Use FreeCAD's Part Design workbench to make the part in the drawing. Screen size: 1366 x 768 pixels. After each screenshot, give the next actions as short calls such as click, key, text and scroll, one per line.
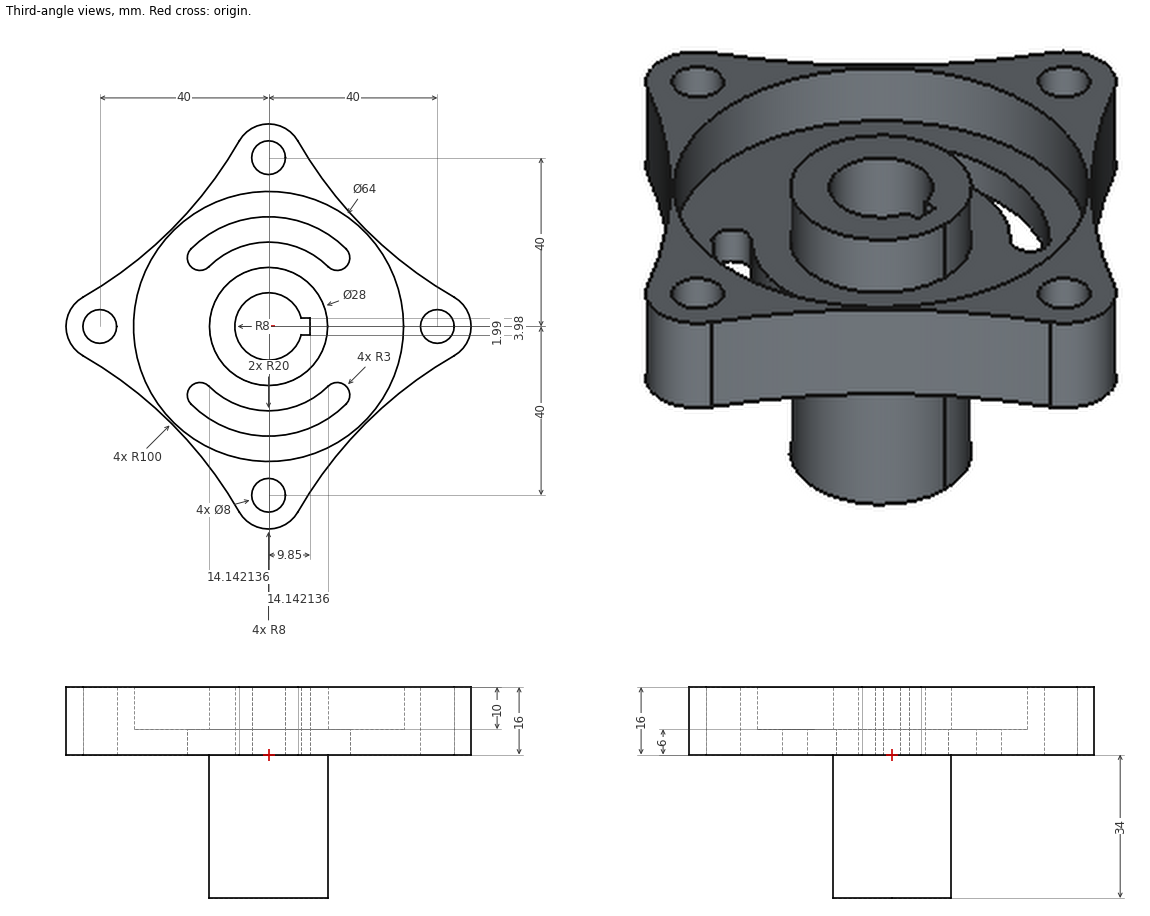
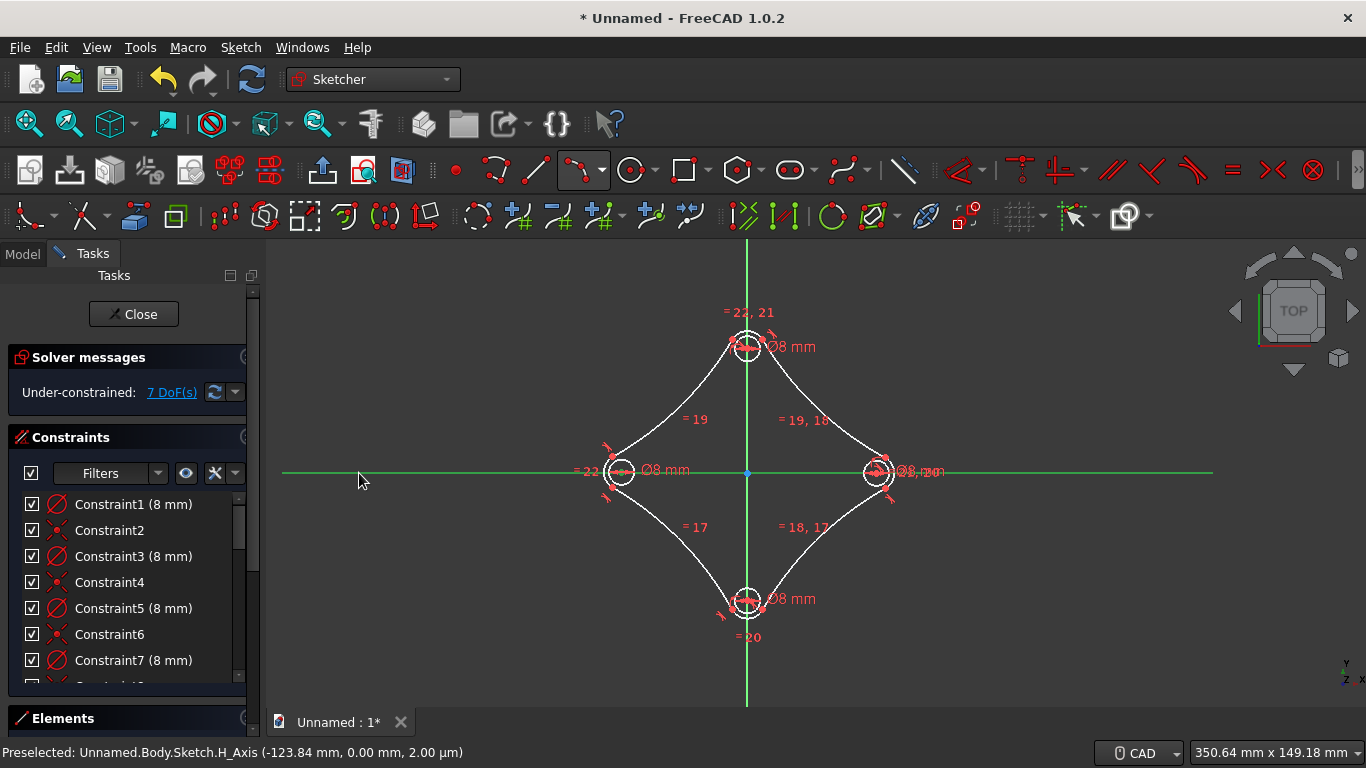
click(1020, 170)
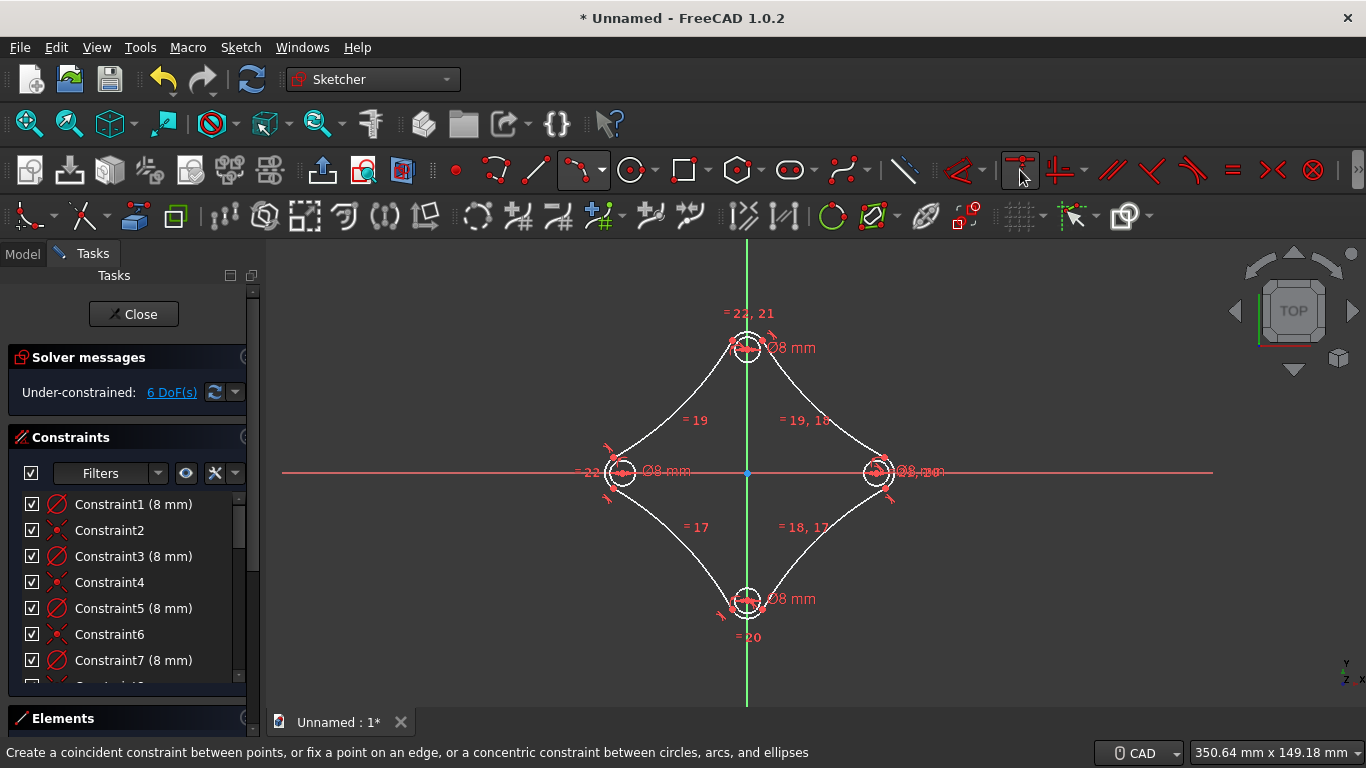
click(958, 170)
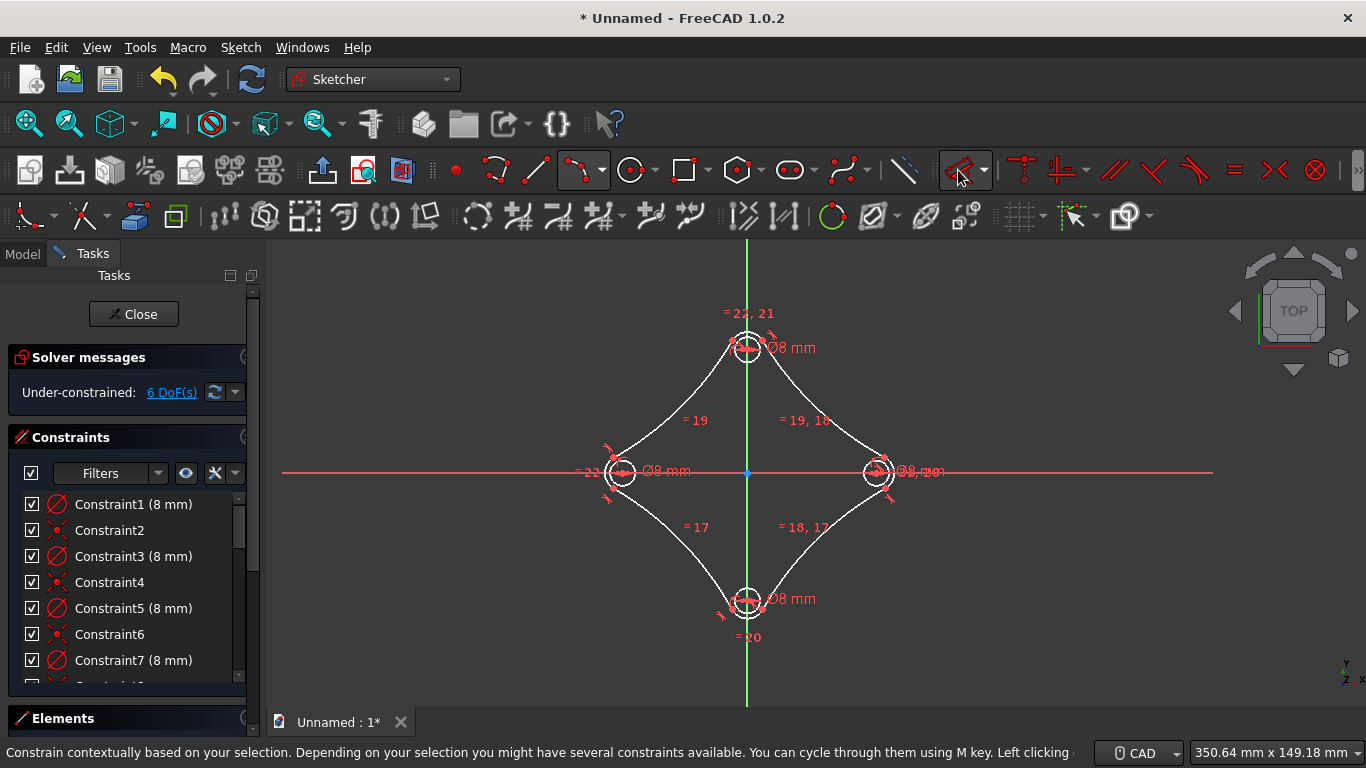
click(704, 567)
click(729, 547)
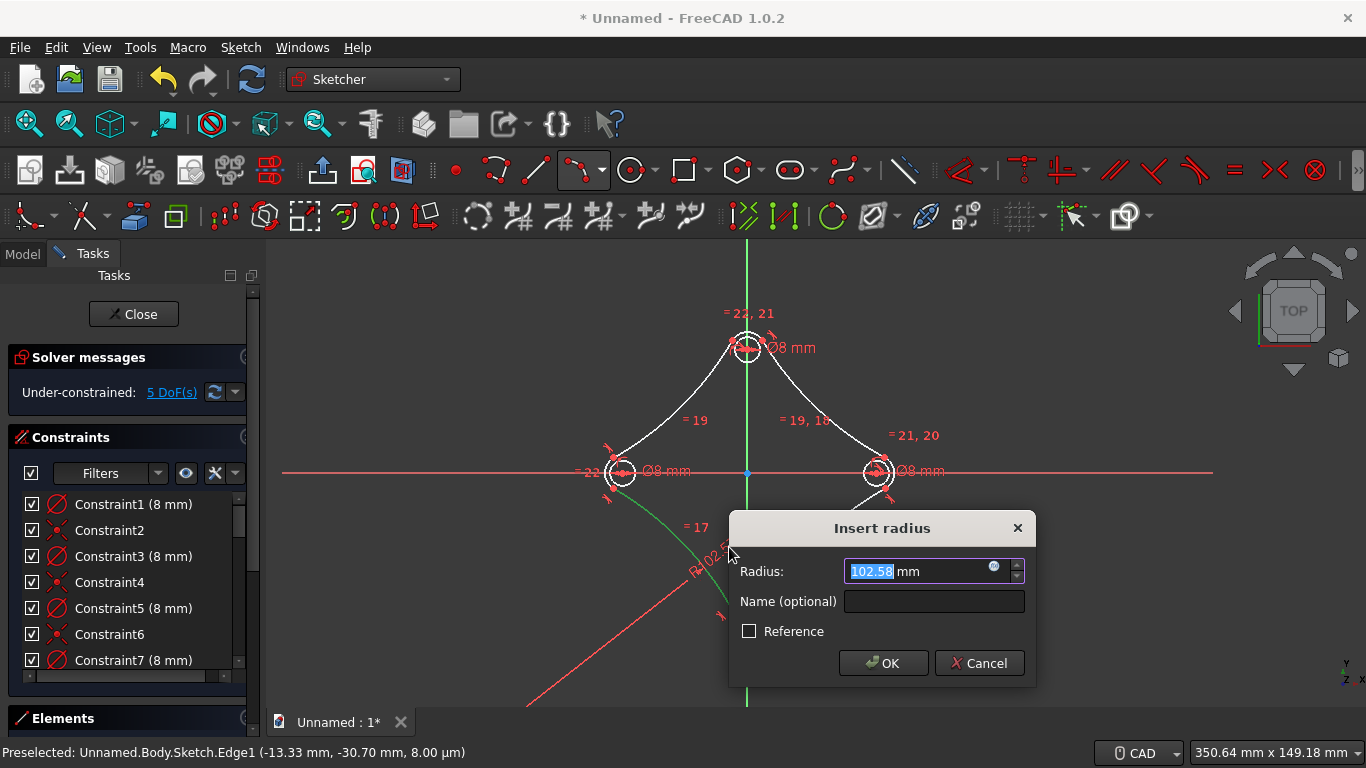
text(100)
key(Return)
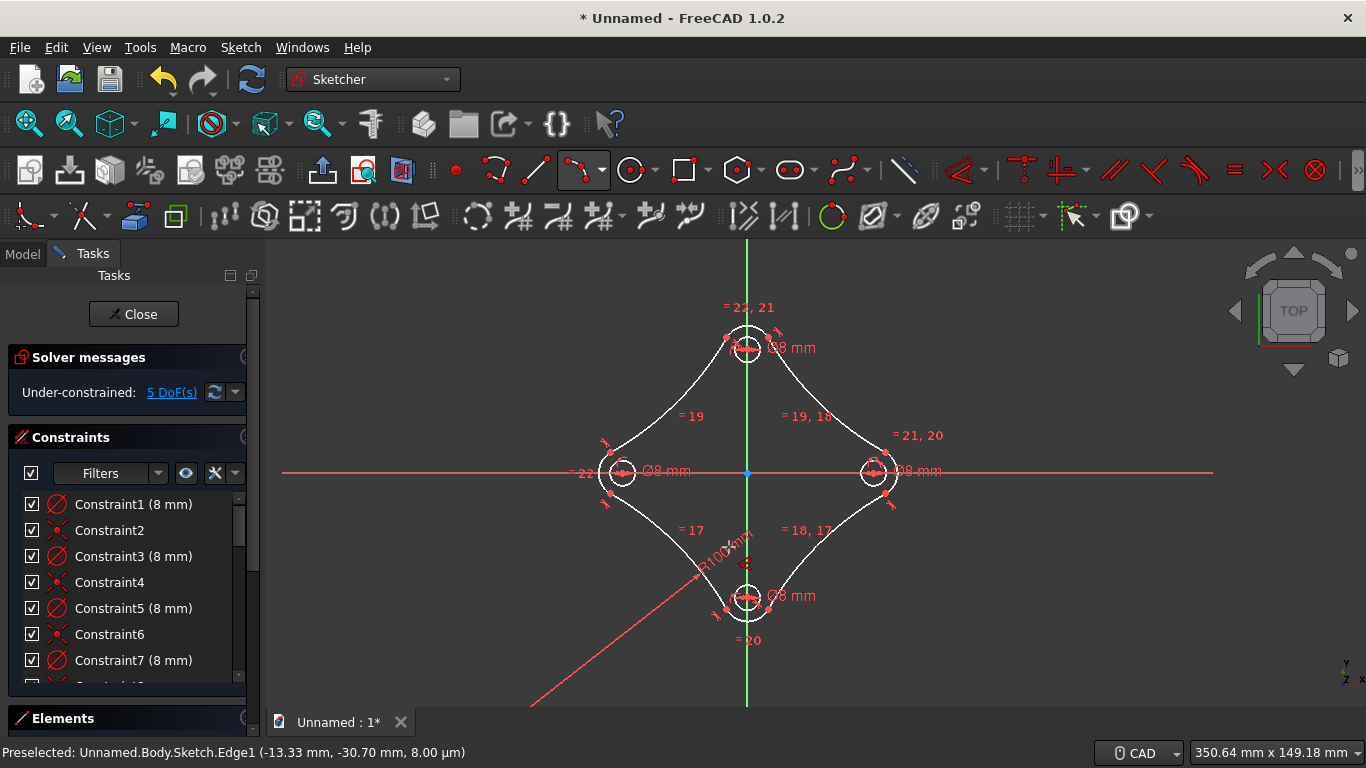
scroll(738, 619, up, 3)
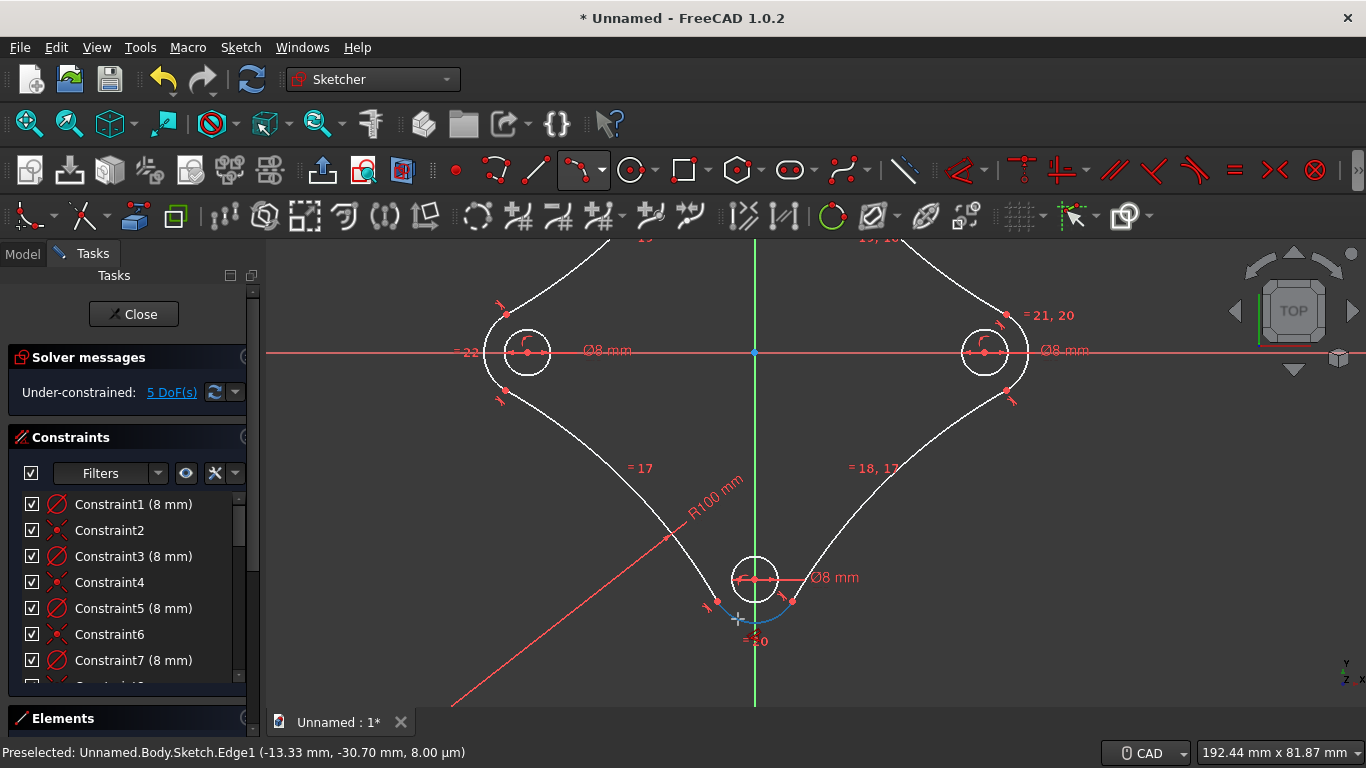
click(737, 619)
click(724, 648)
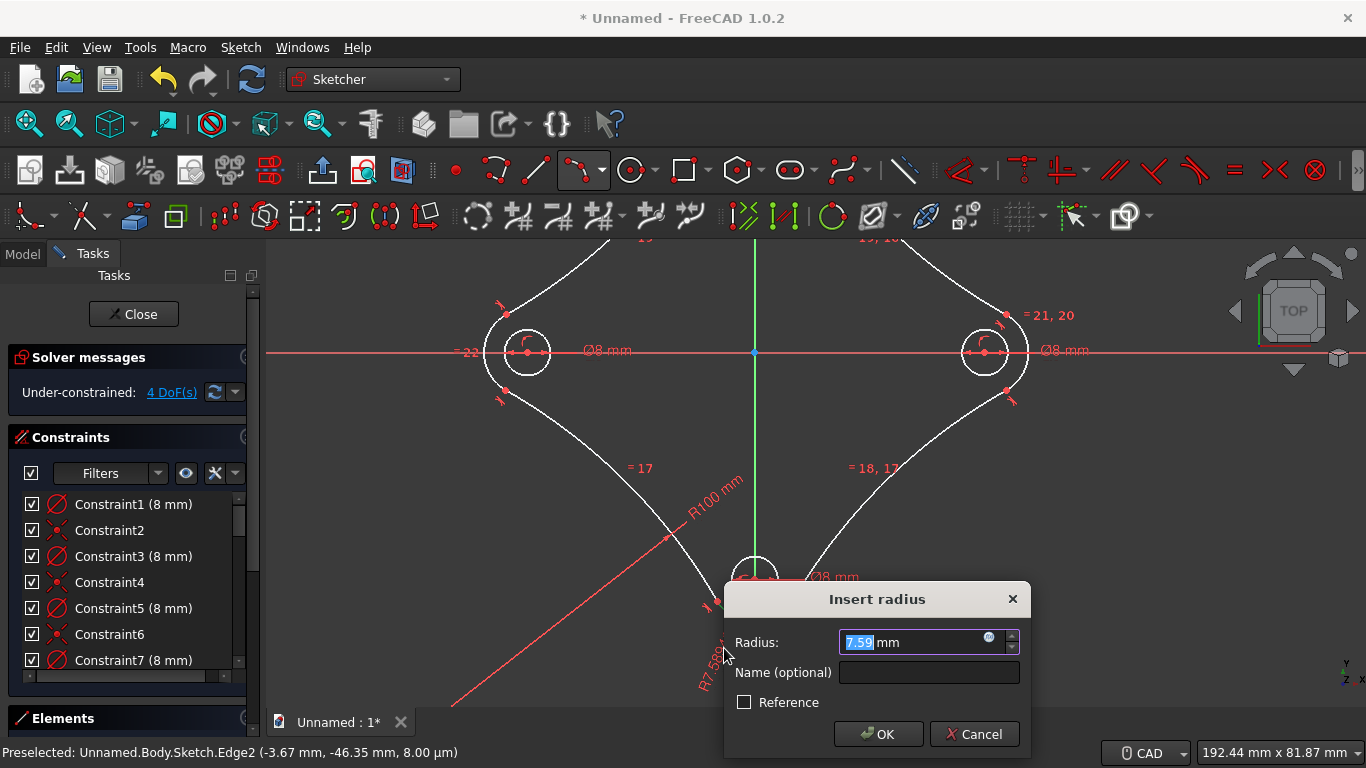
text(8)
key(Return)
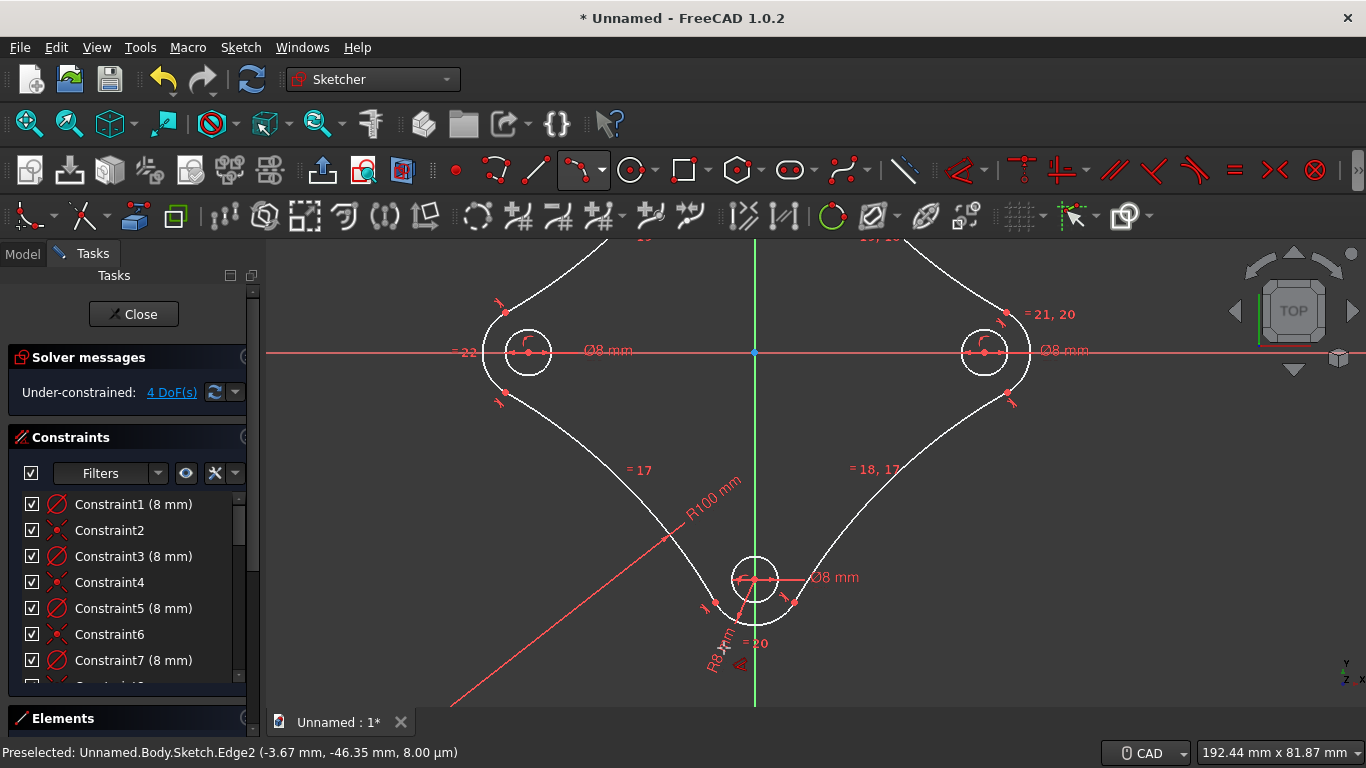
click(755, 580)
click(789, 466)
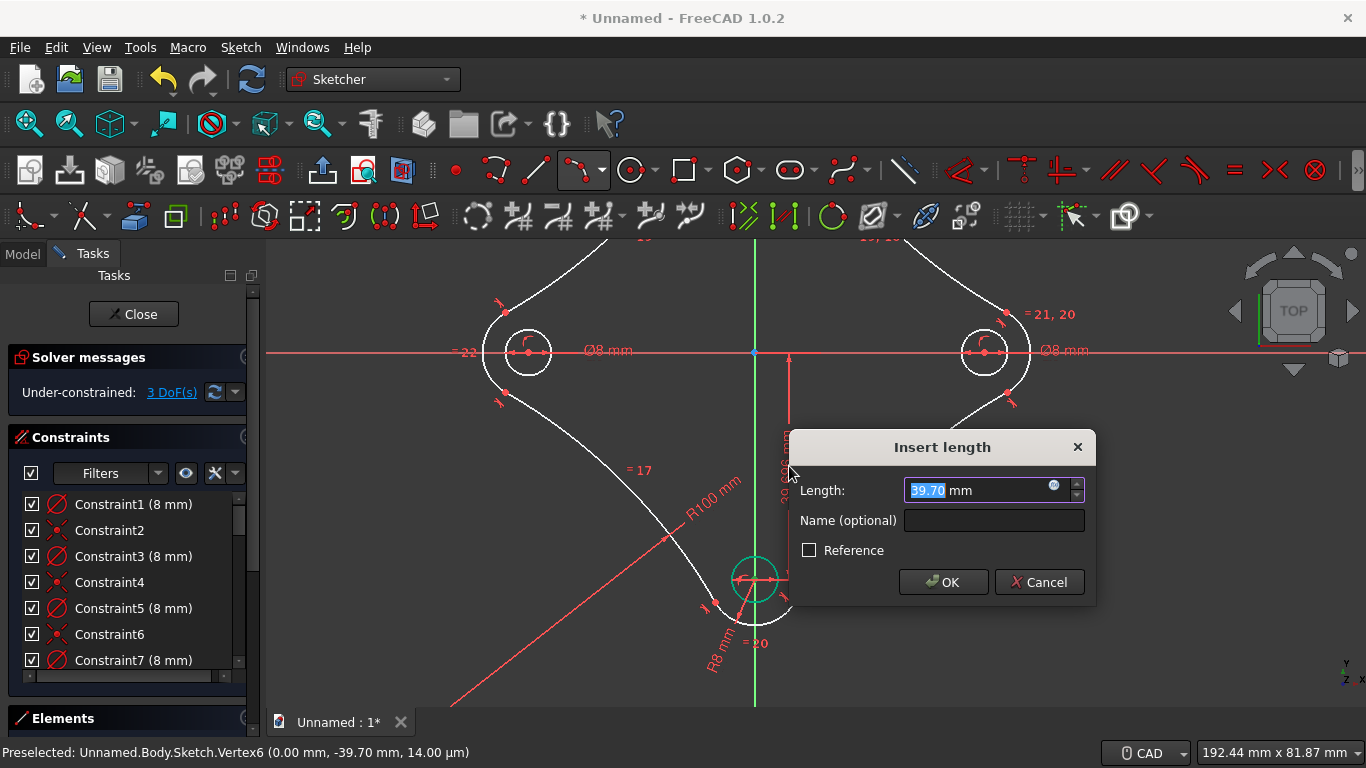
text(40)
key(Return)